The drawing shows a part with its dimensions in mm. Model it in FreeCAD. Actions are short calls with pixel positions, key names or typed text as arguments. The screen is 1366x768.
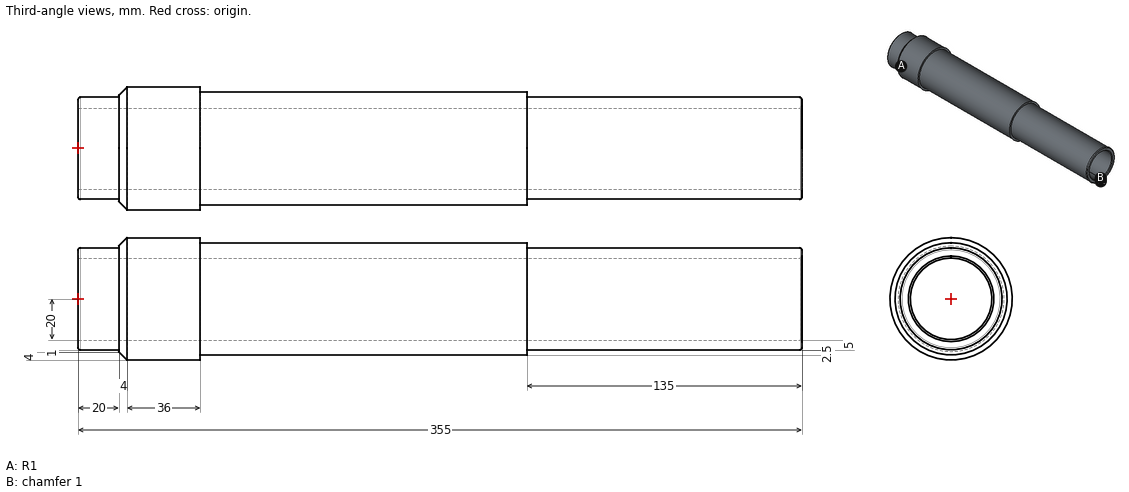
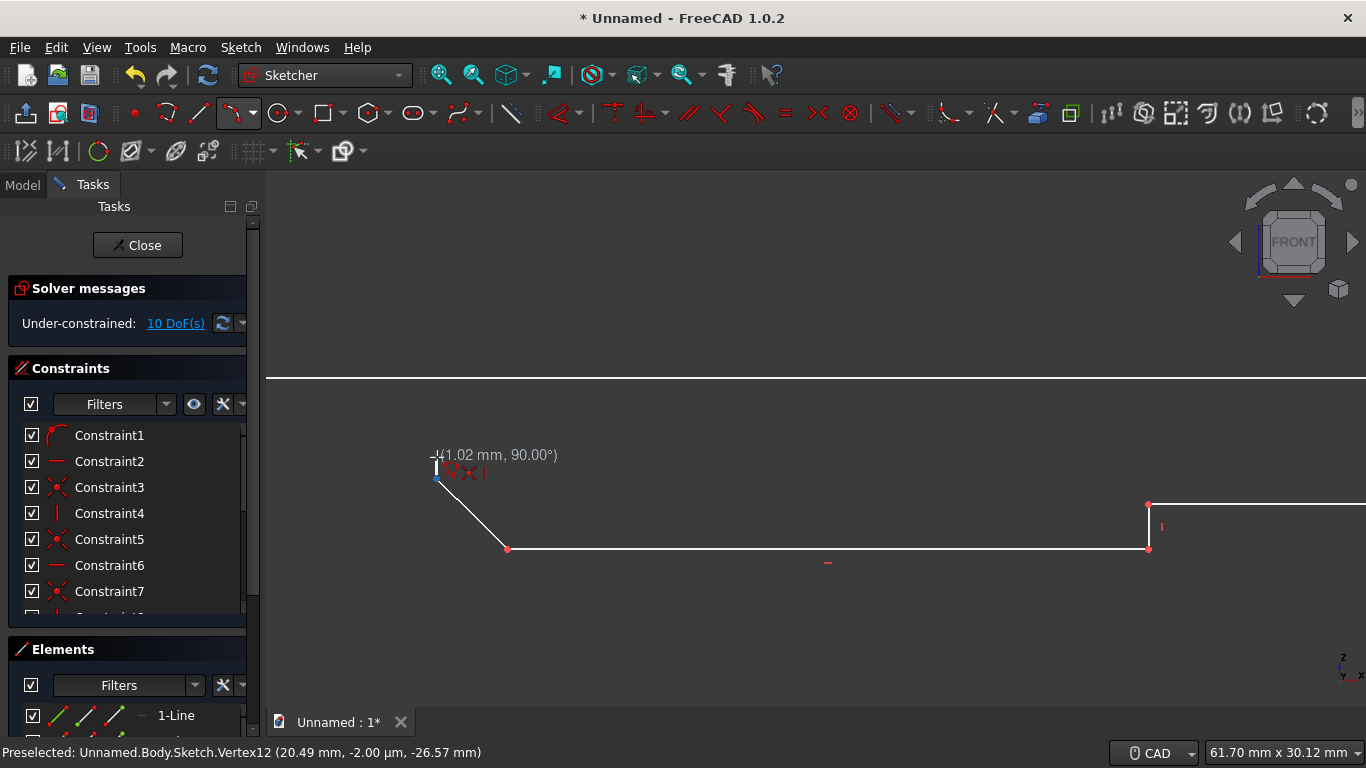
click(436, 456)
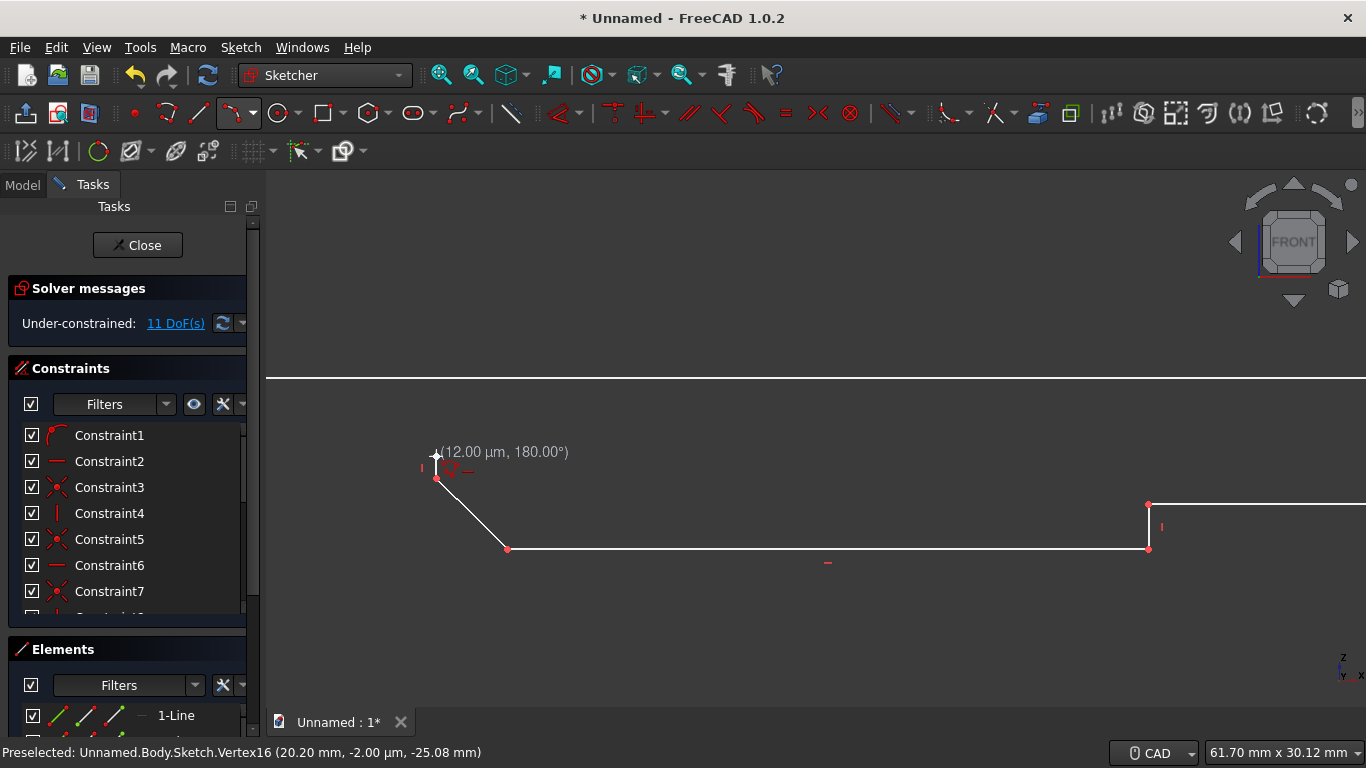
scroll(437, 458, down, 11)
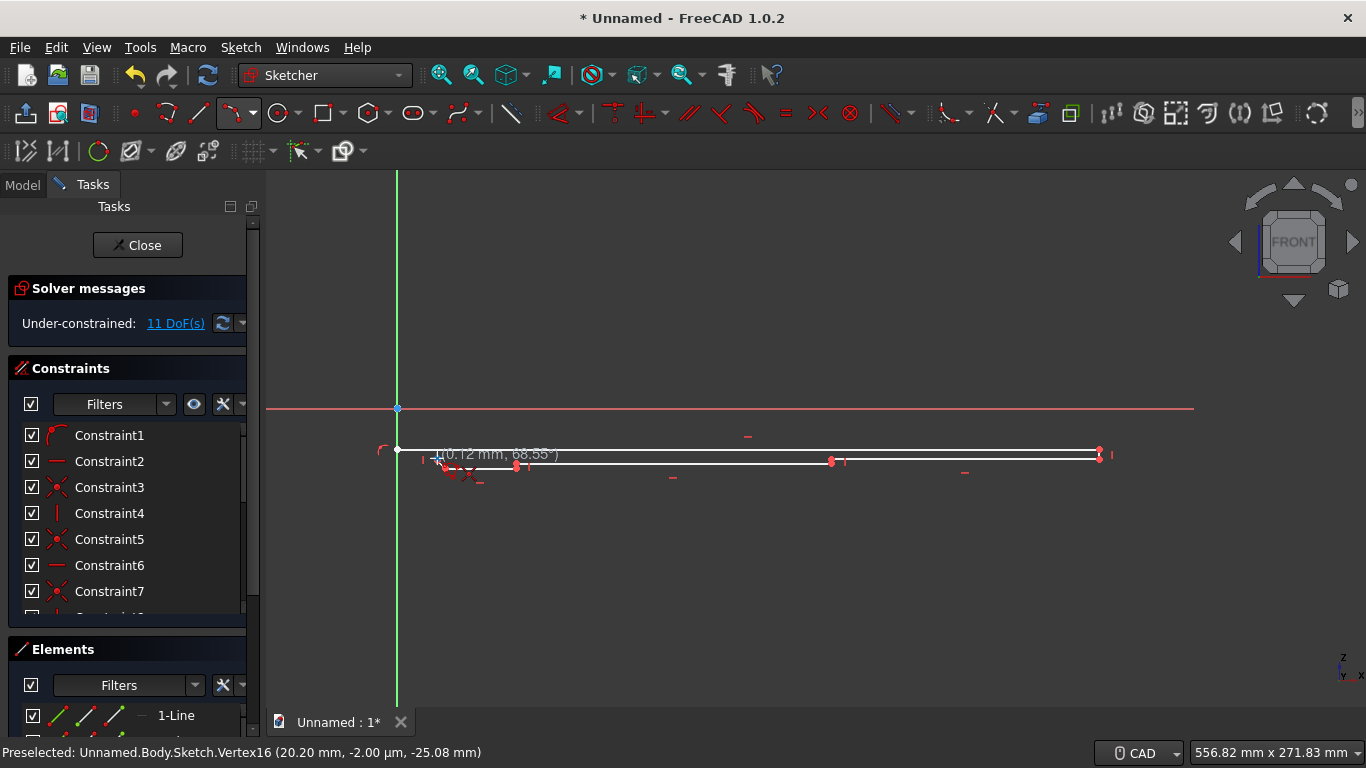
scroll(397, 458, up, 3)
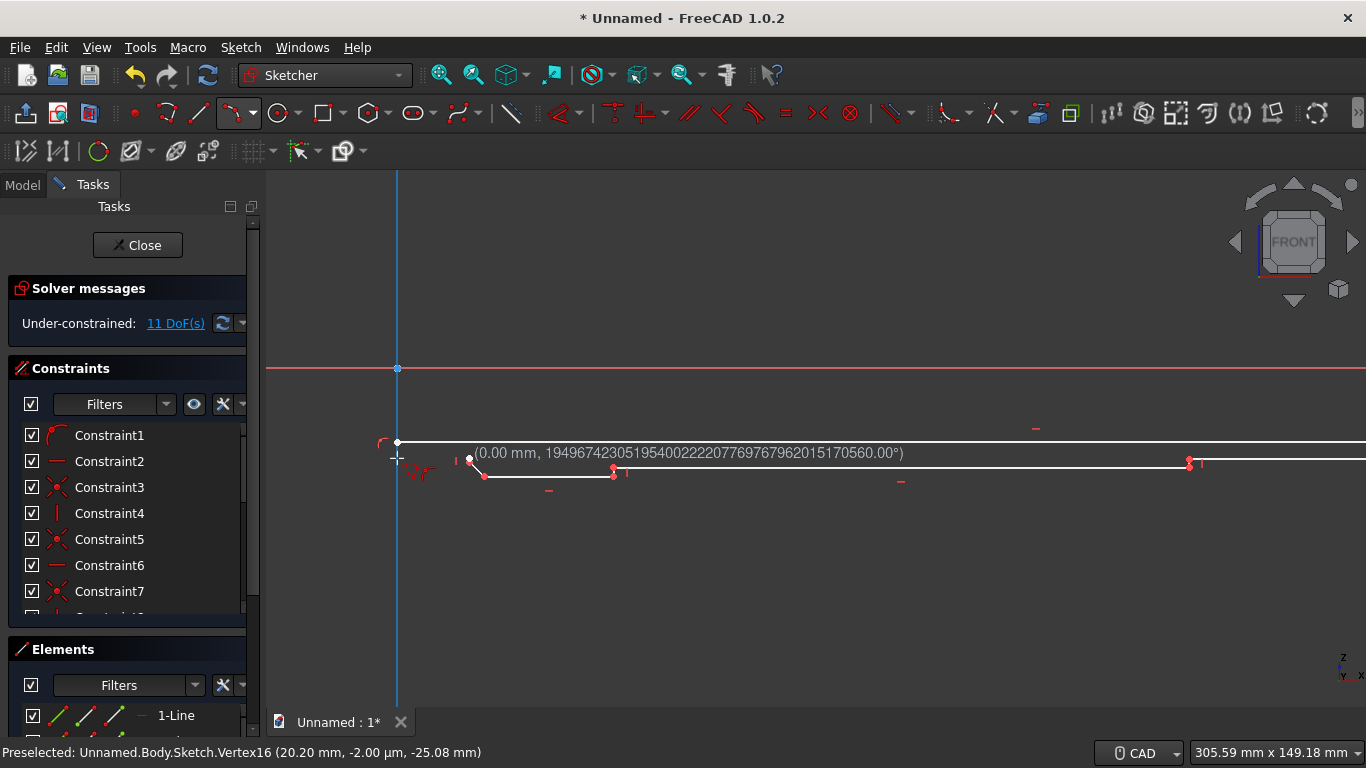
click(406, 458)
click(397, 442)
key(Escape)
key(Escape)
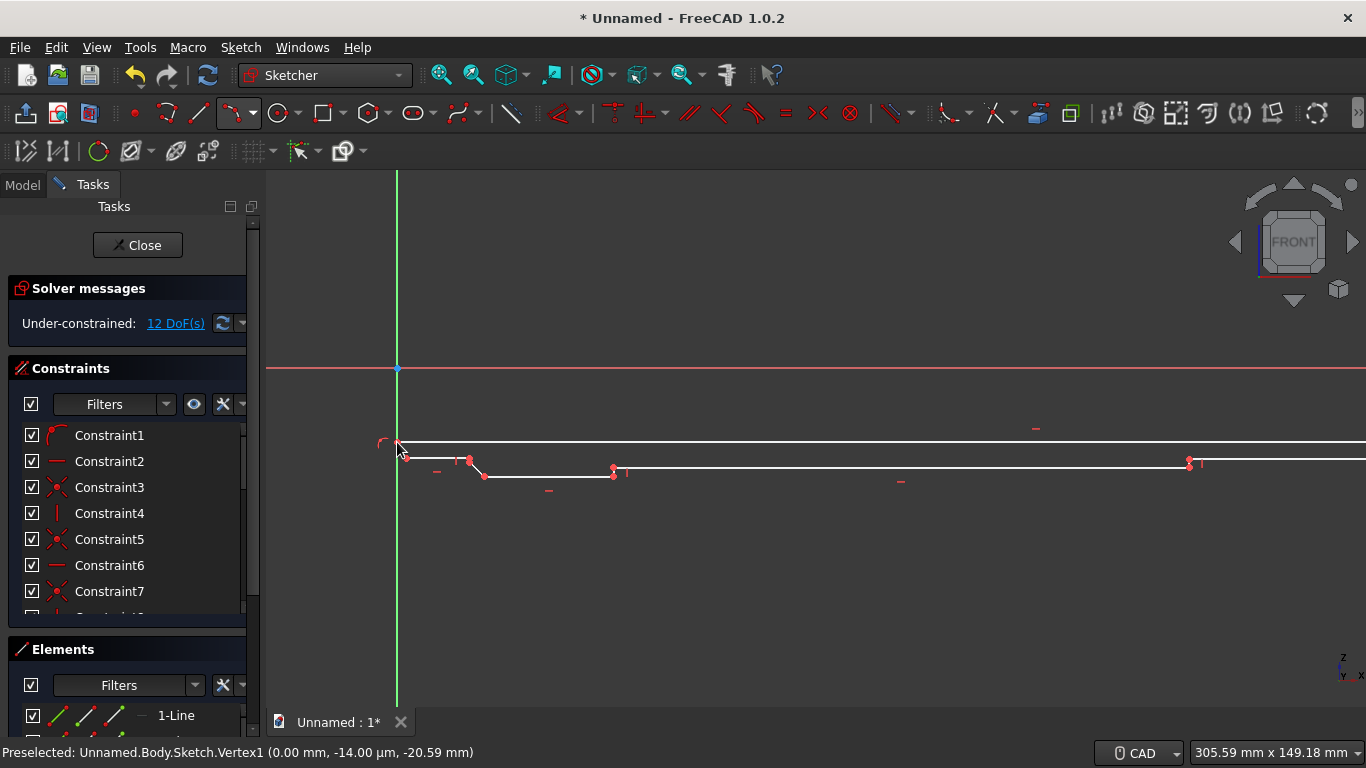
scroll(401, 449, up, 4)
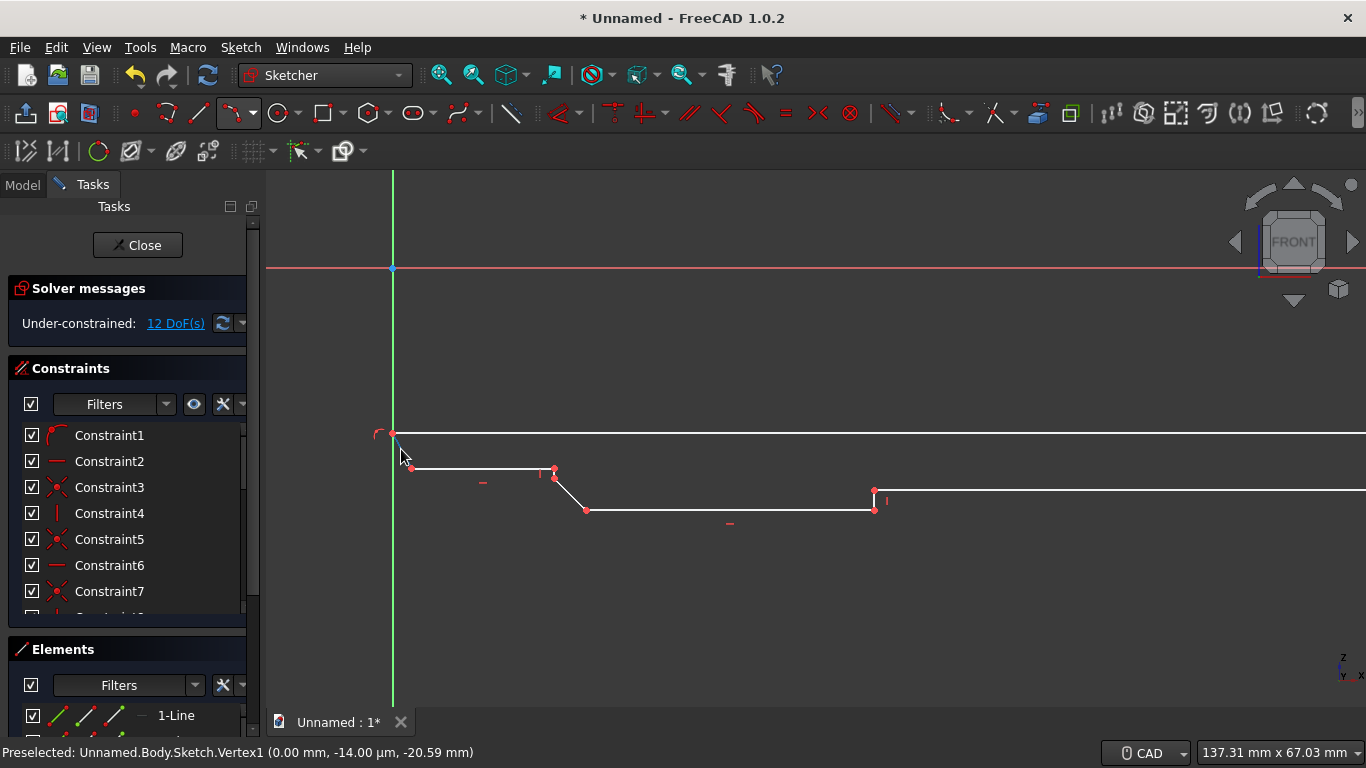
click(400, 448)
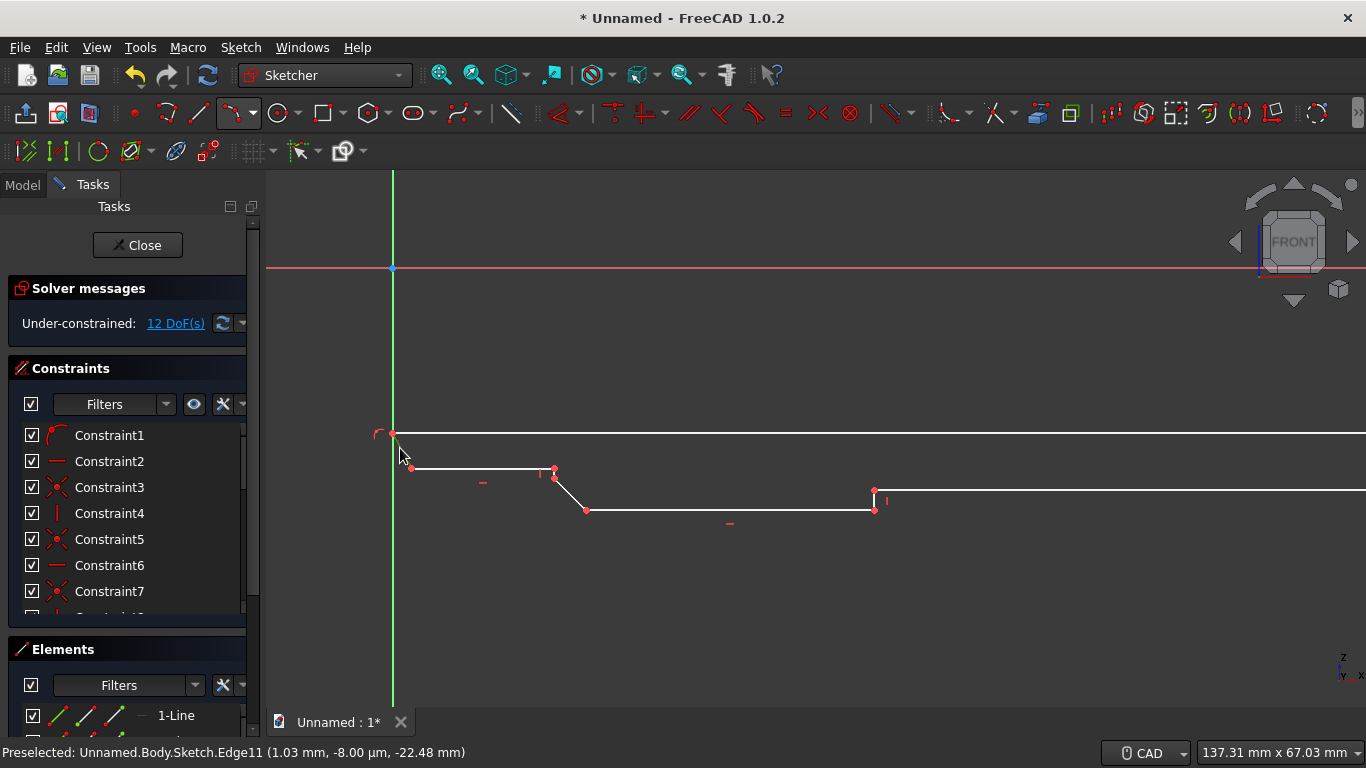
key(v)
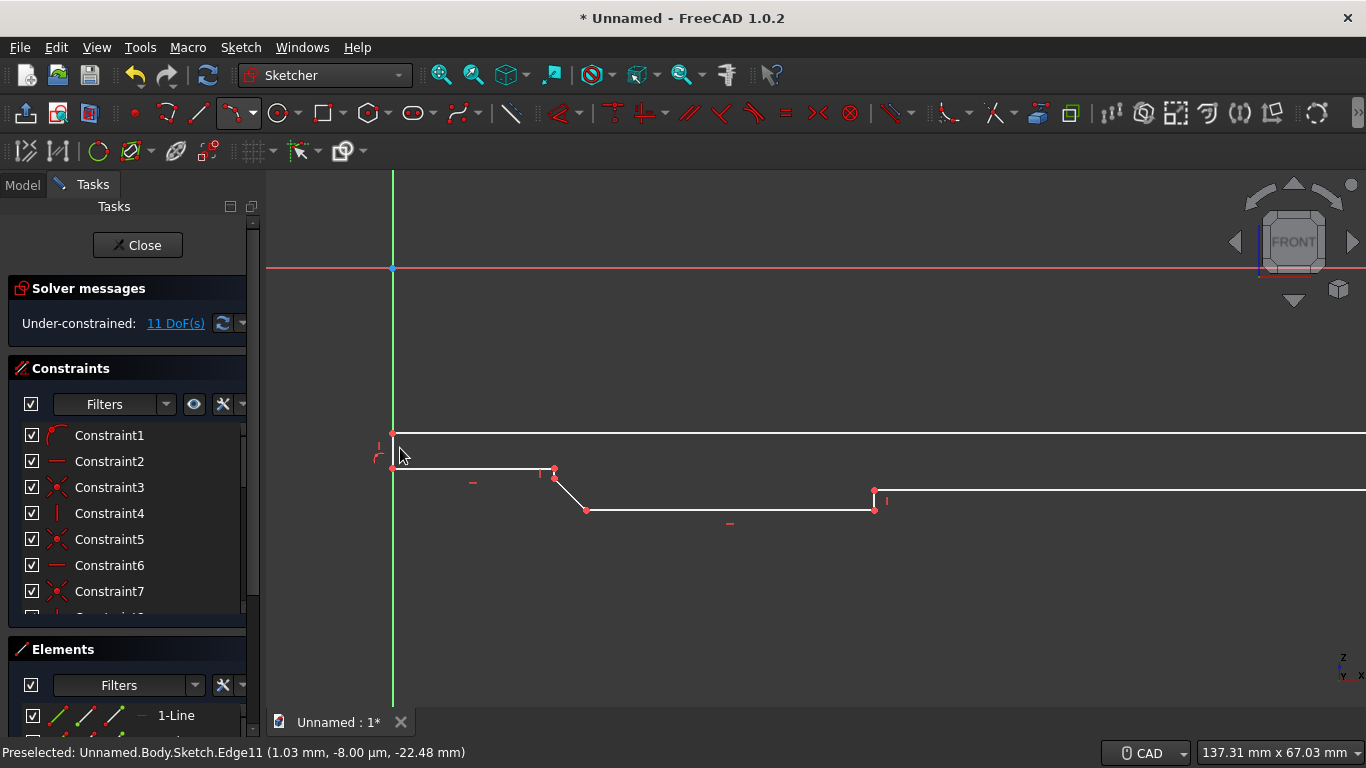
click(558, 114)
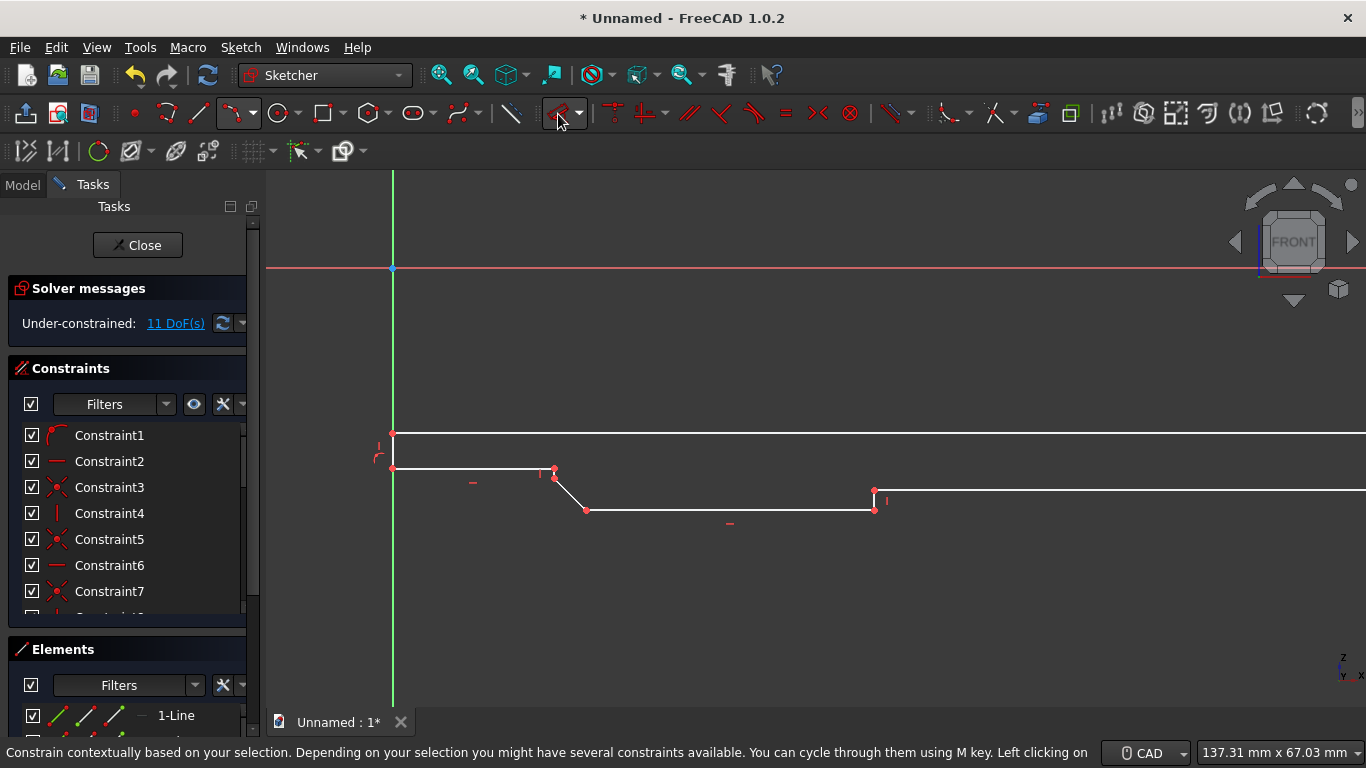
scroll(398, 455, down, 7)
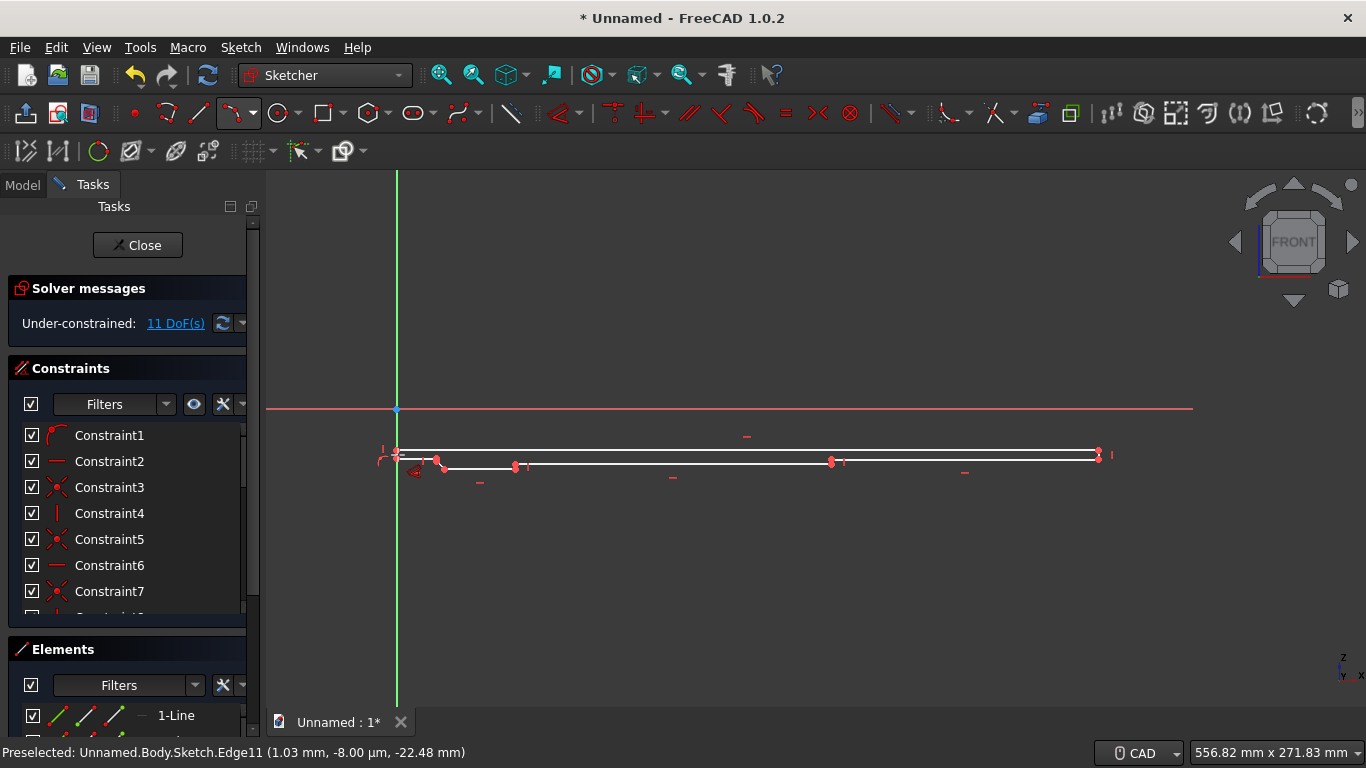
scroll(1099, 453, up, 8)